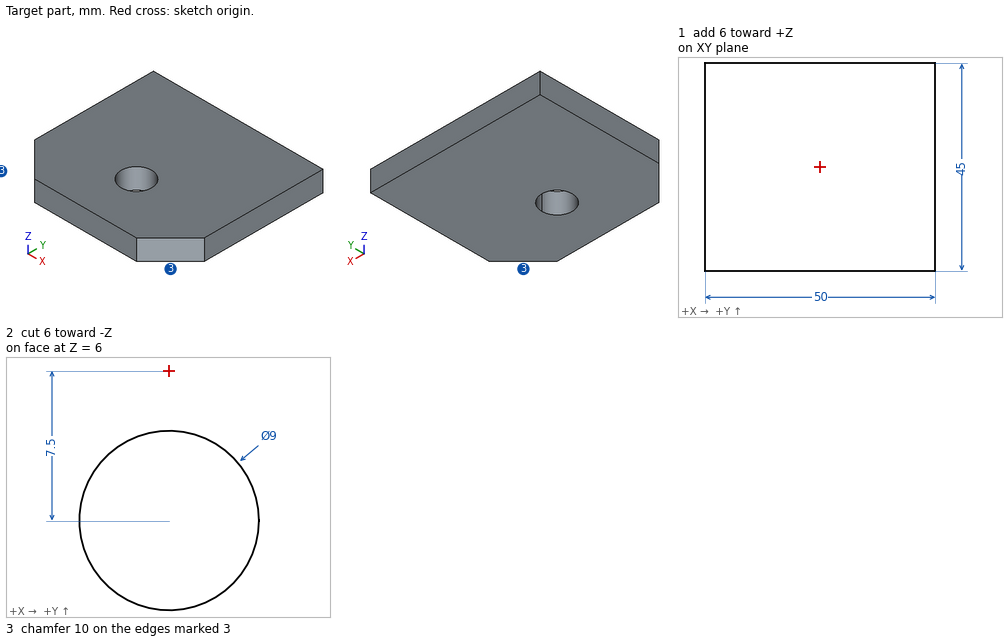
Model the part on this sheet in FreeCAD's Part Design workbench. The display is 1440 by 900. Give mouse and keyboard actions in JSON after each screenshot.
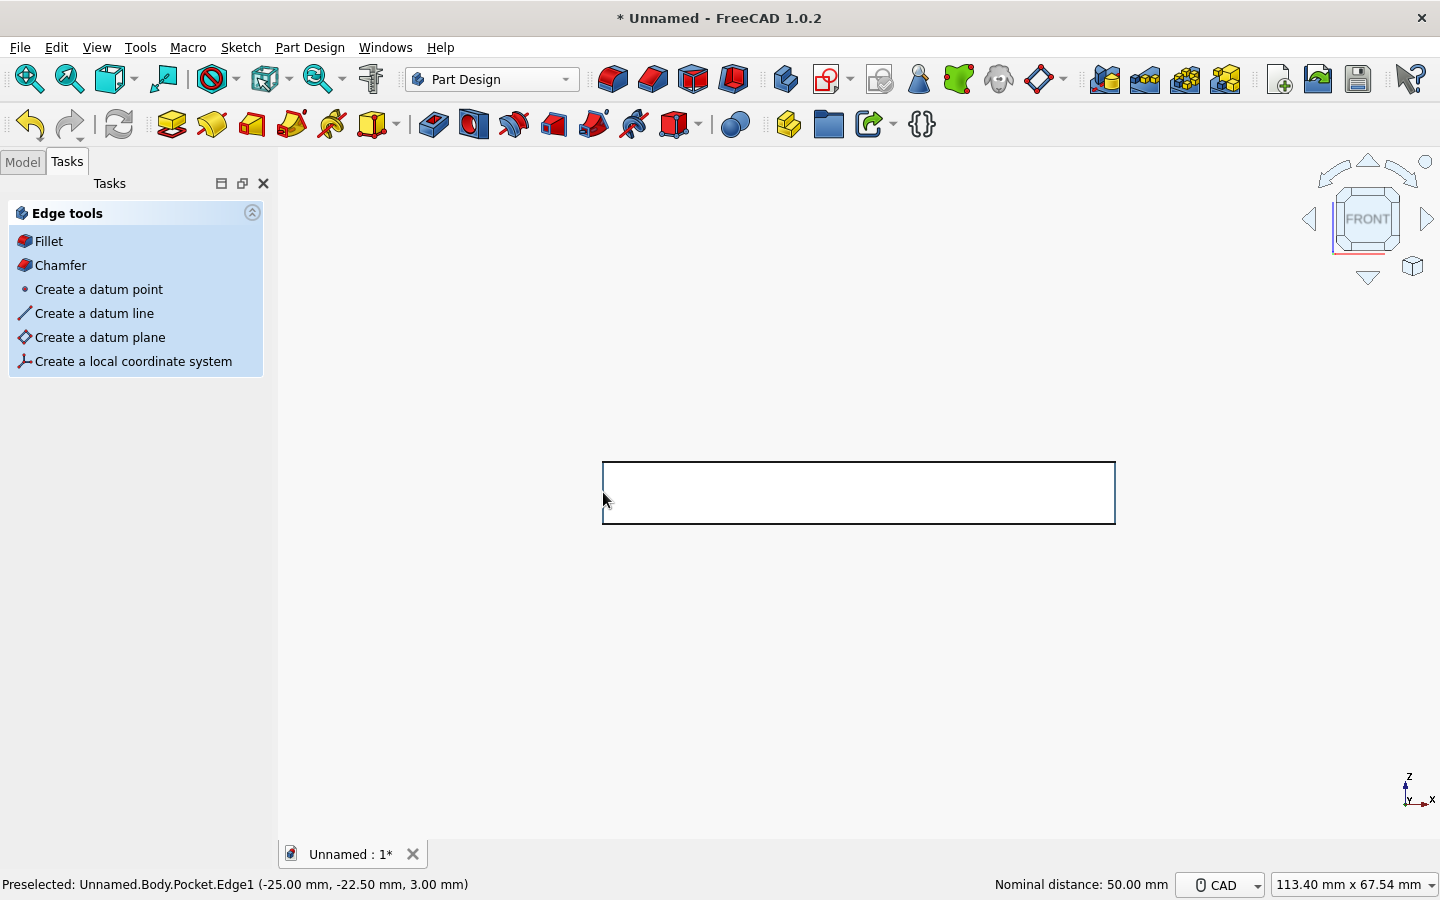
{"action": "left_click", "coordinate": [654, 80]}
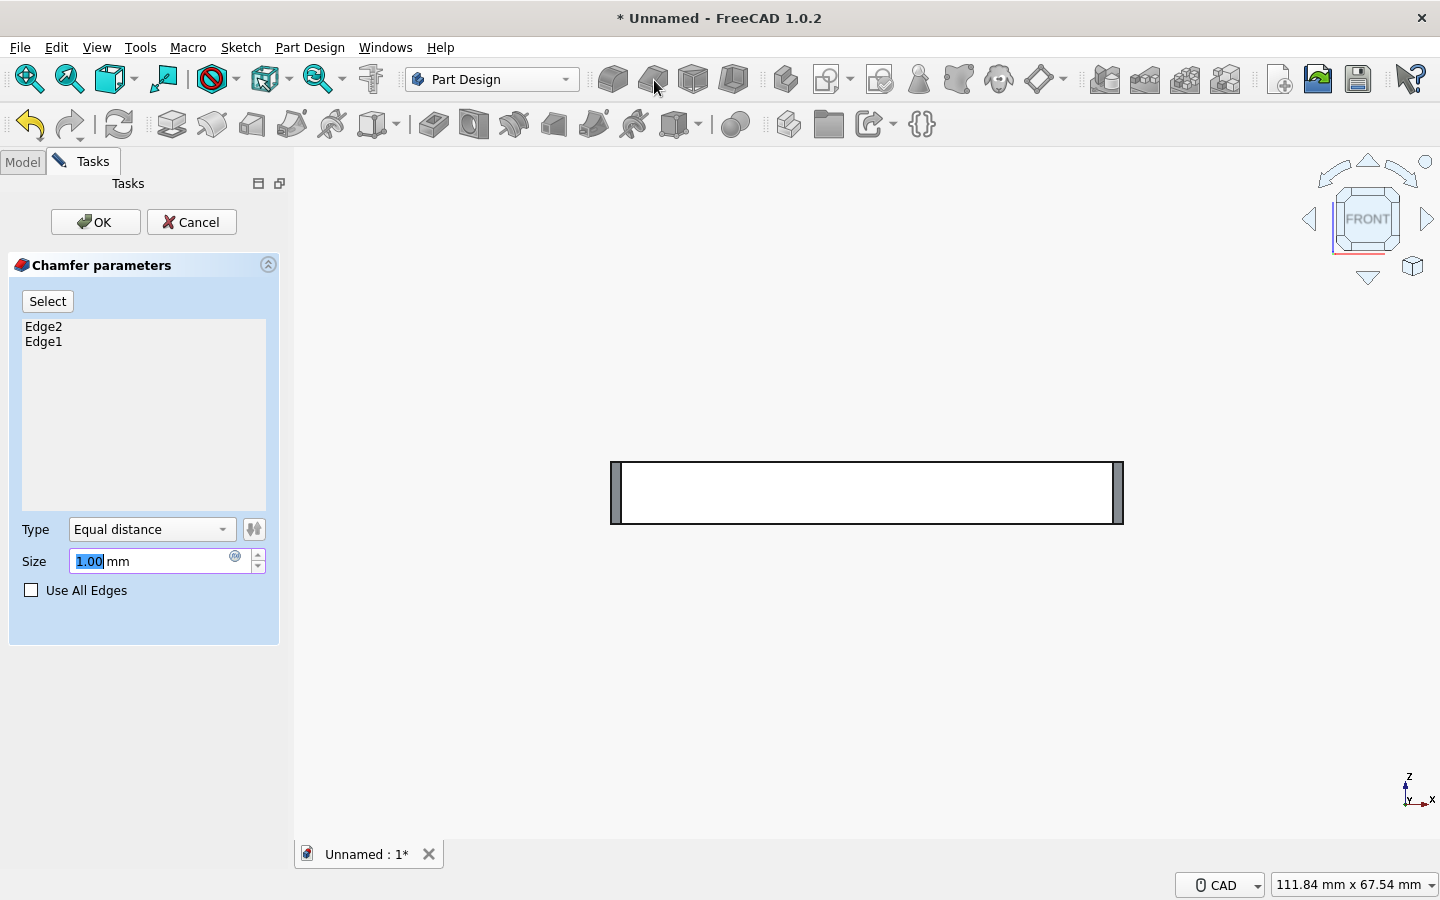
{"action": "type", "text": "10"}
{"action": "key", "text": "Tab"}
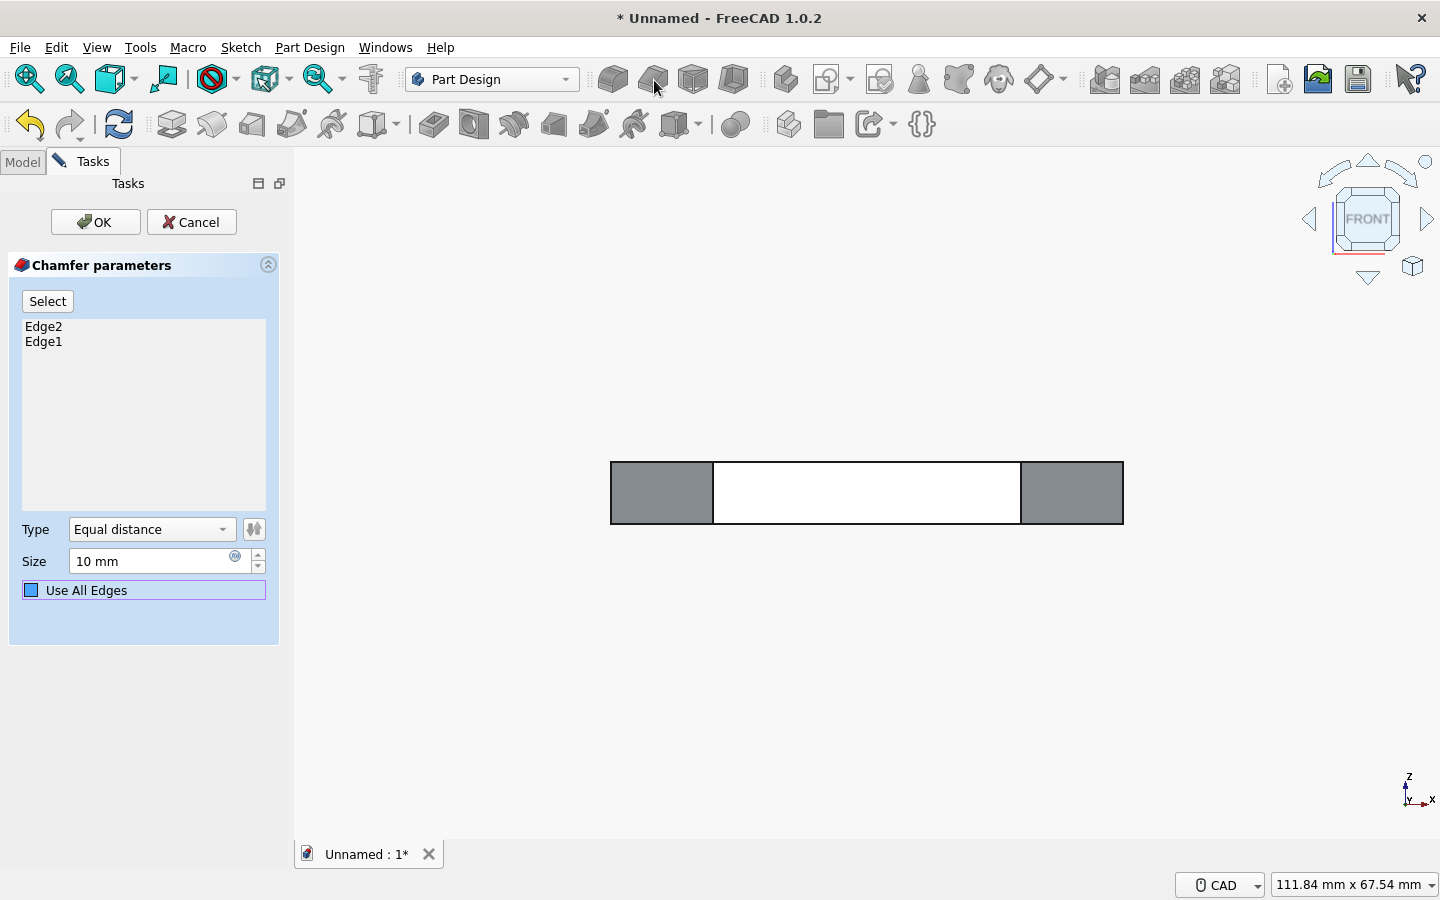
{"action": "left_click", "coordinate": [96, 222]}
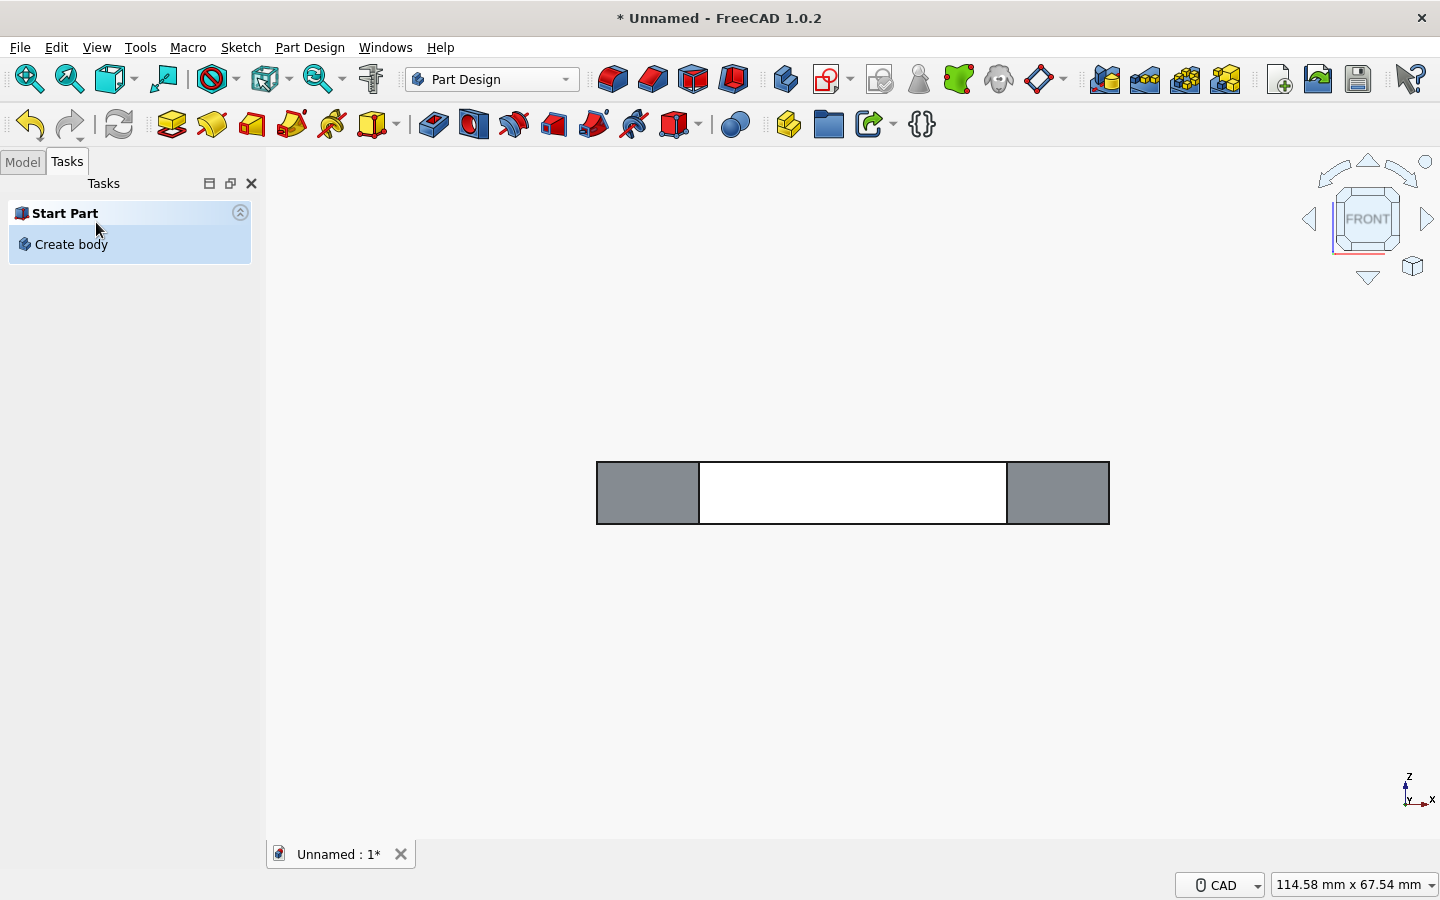
{"action": "key", "text": "0"}